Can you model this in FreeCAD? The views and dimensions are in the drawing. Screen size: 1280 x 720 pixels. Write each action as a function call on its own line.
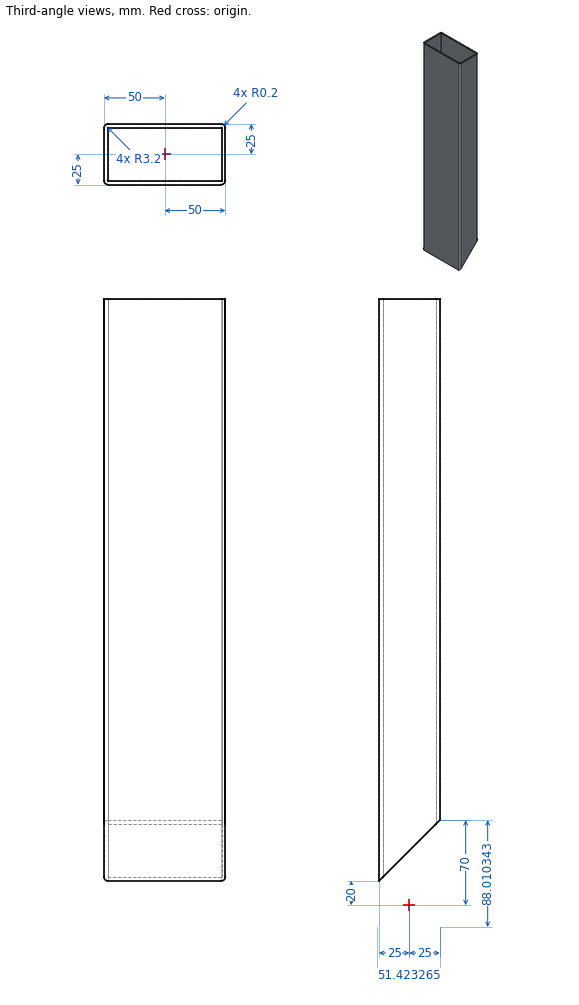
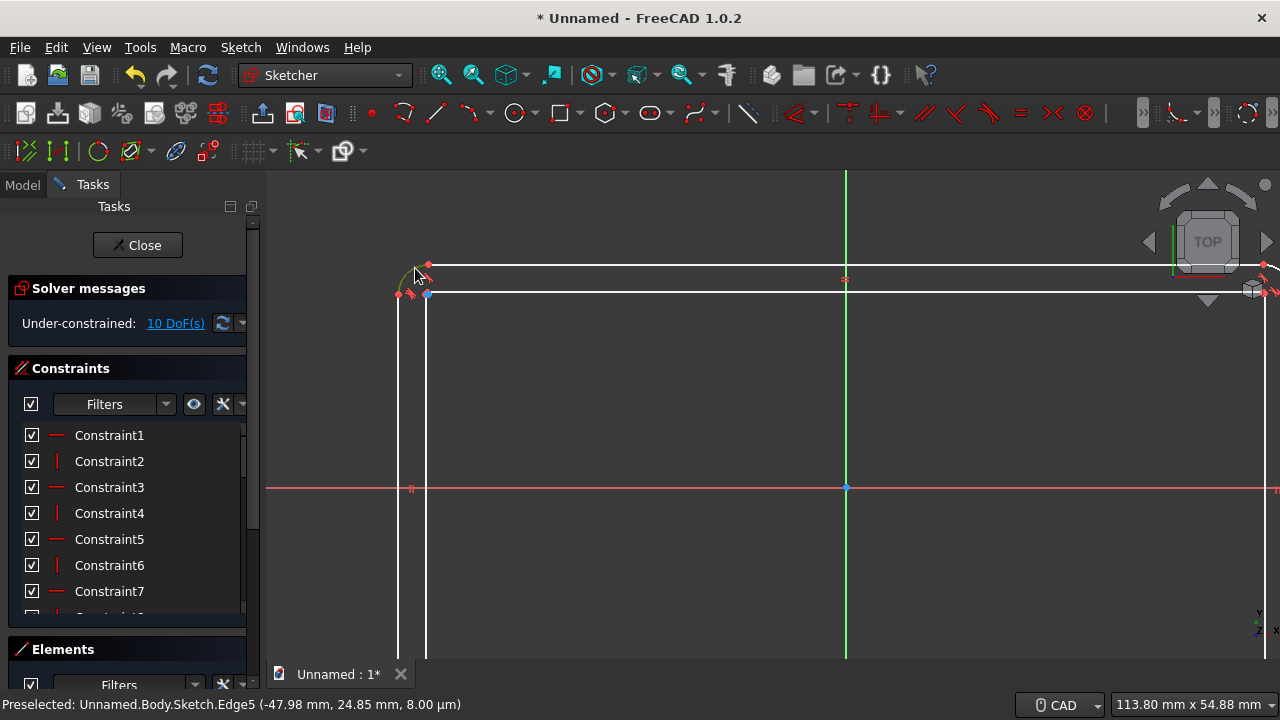
scroll(416, 265, down, 2)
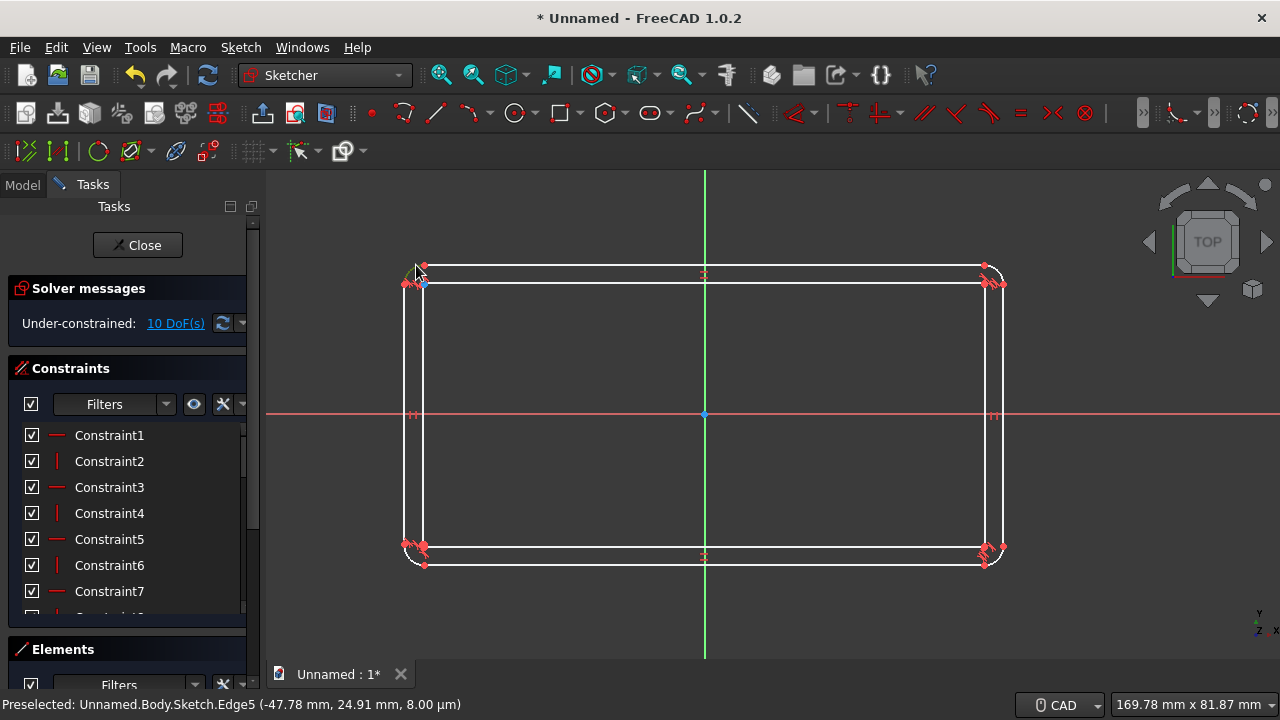
scroll(407, 554, up, 2)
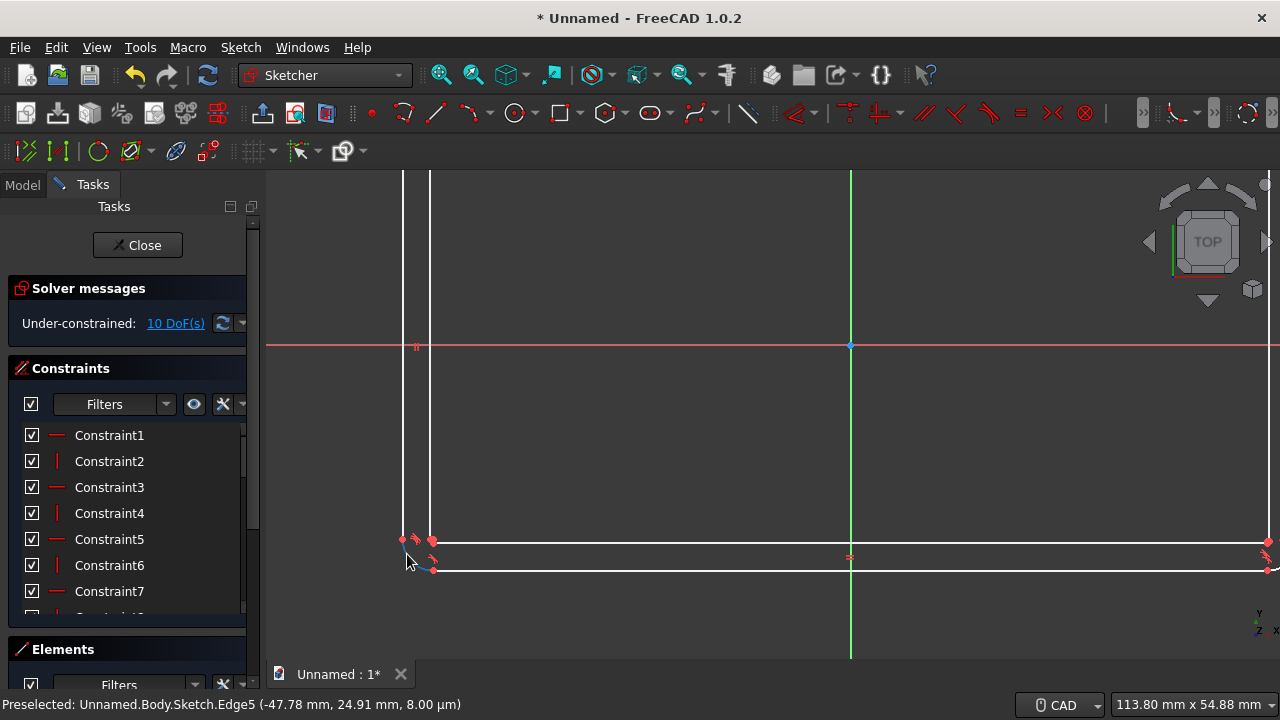
click(406, 554)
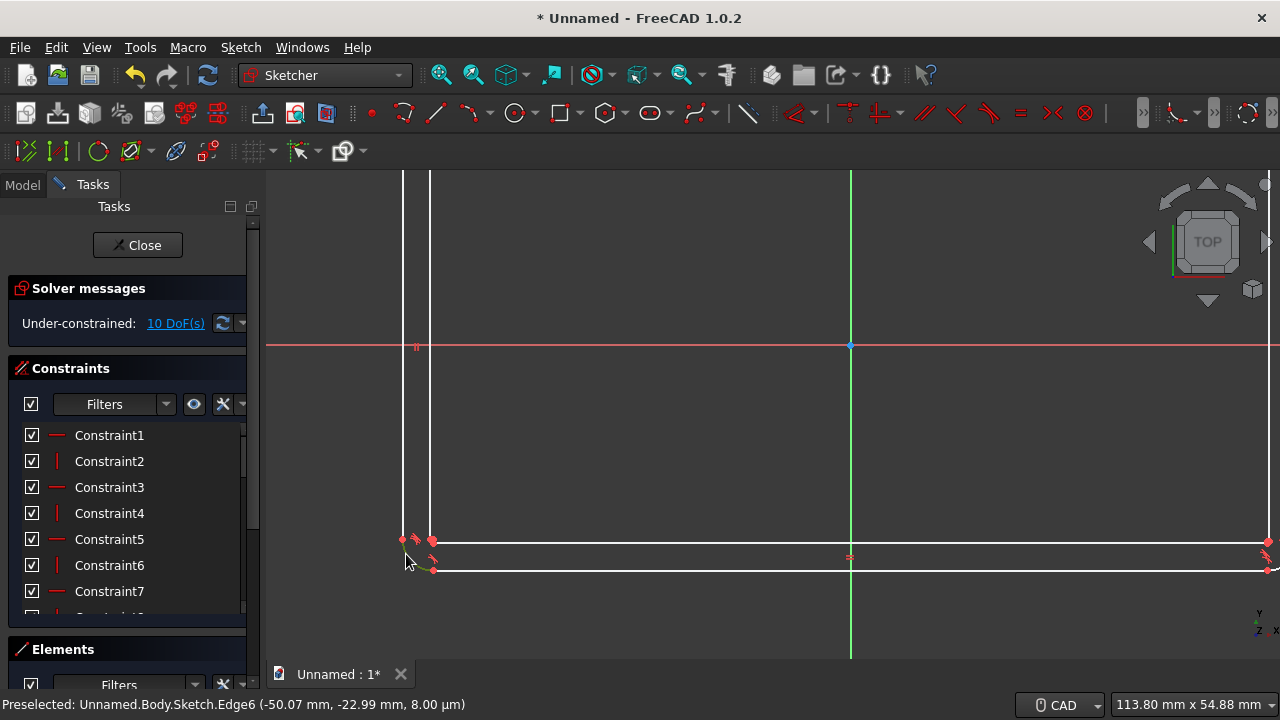
scroll(407, 555, down, 2)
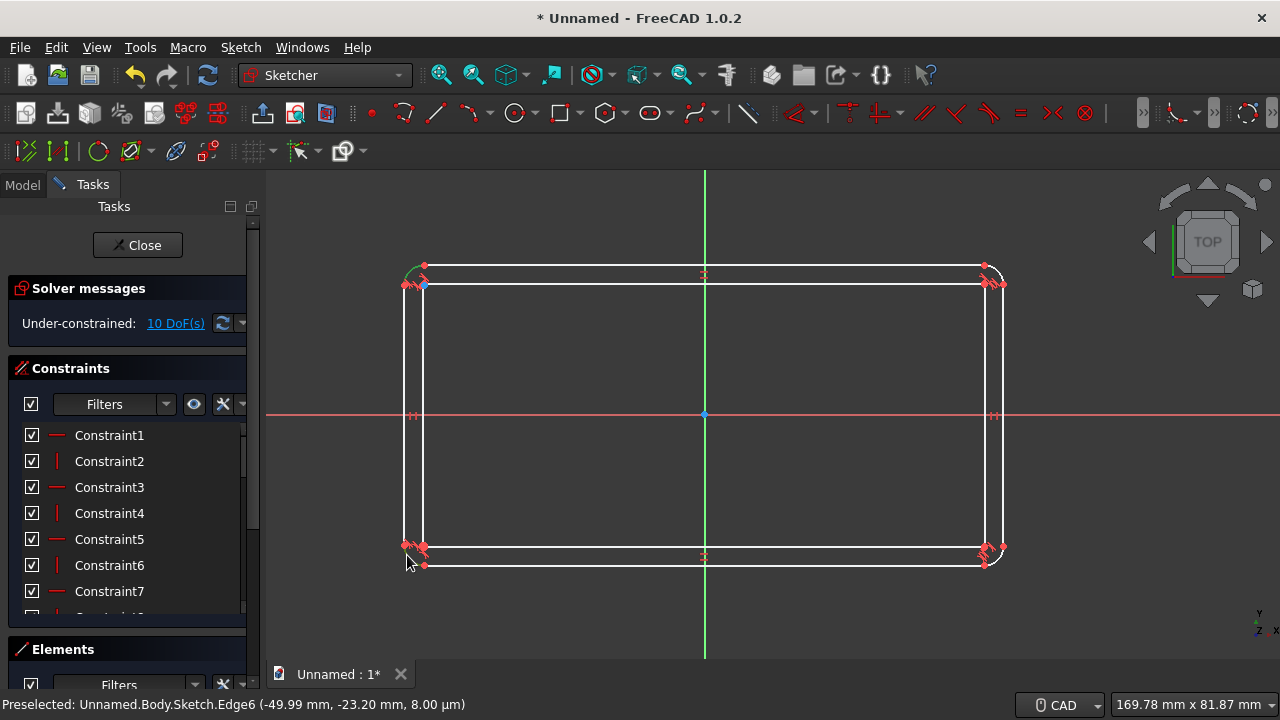
scroll(993, 564, up, 3)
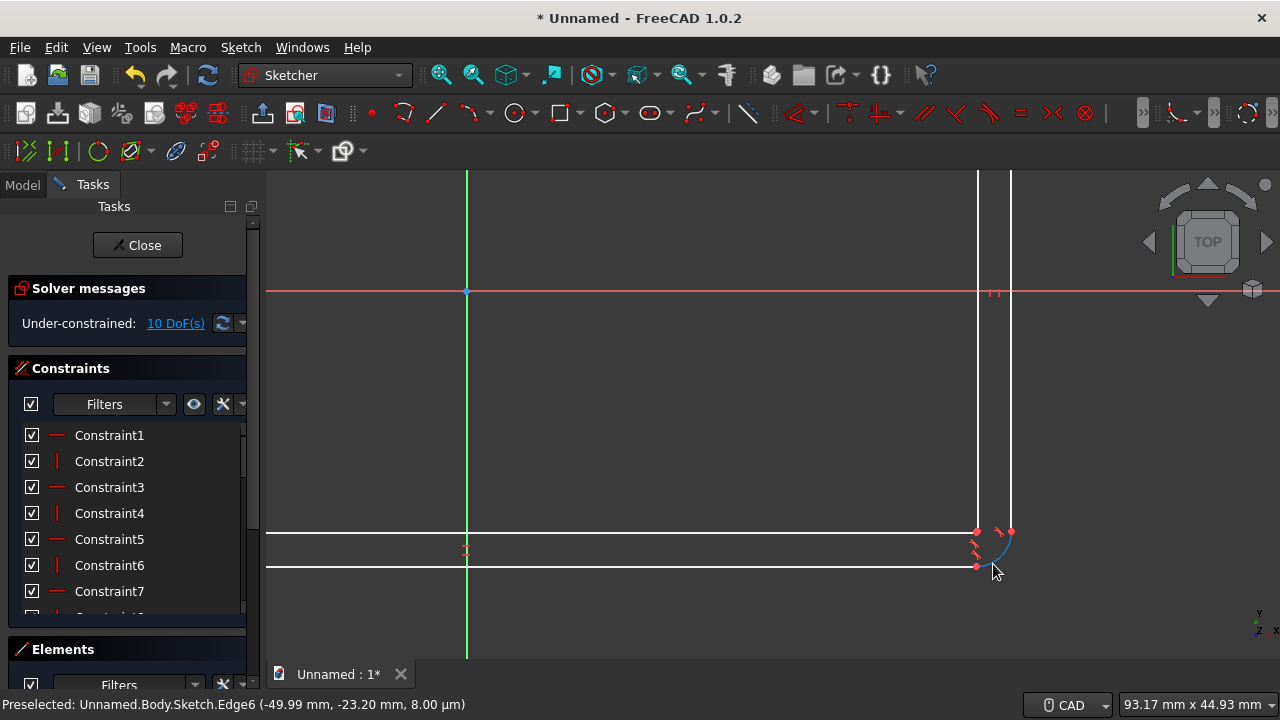
click(992, 563)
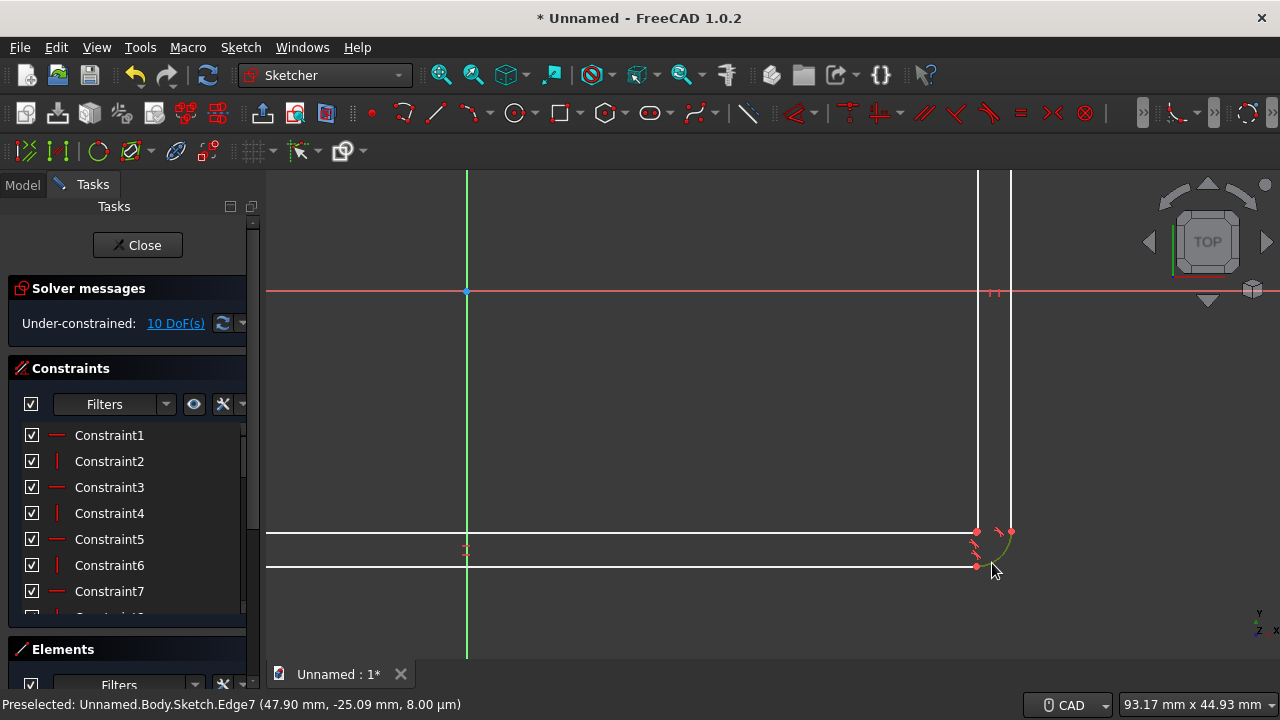
scroll(994, 564, down, 3)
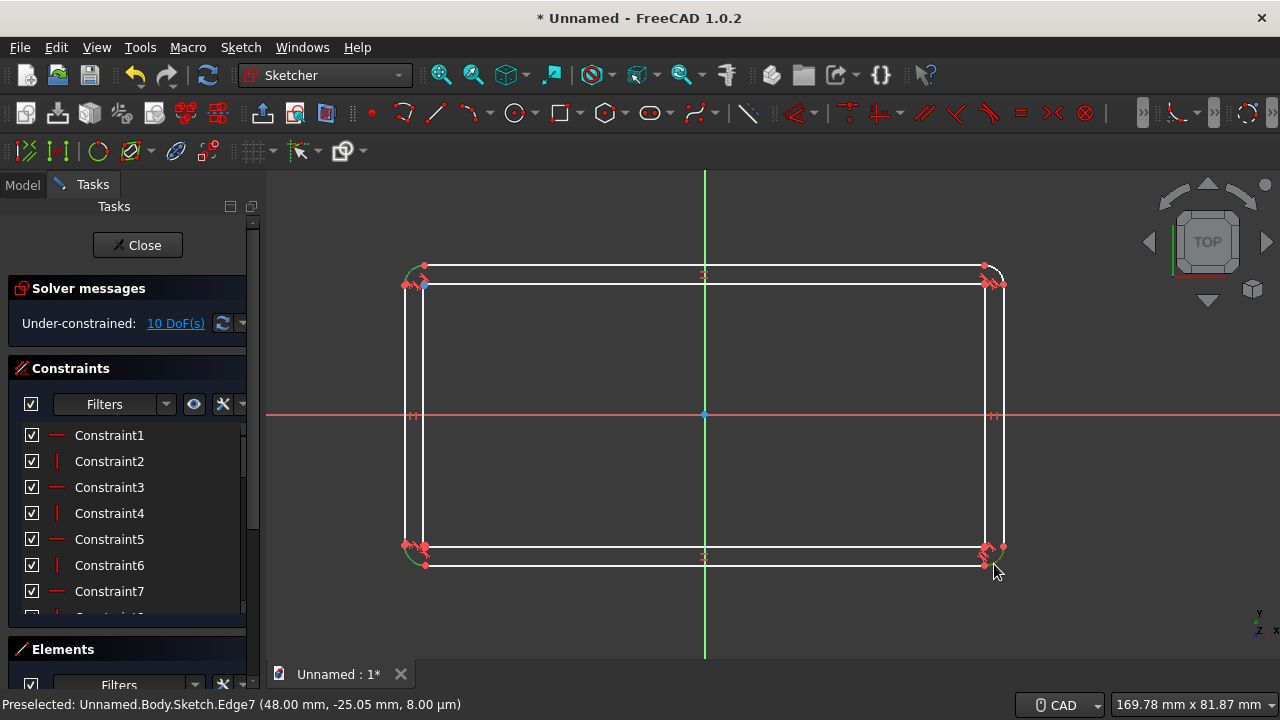
scroll(1002, 276, up, 3)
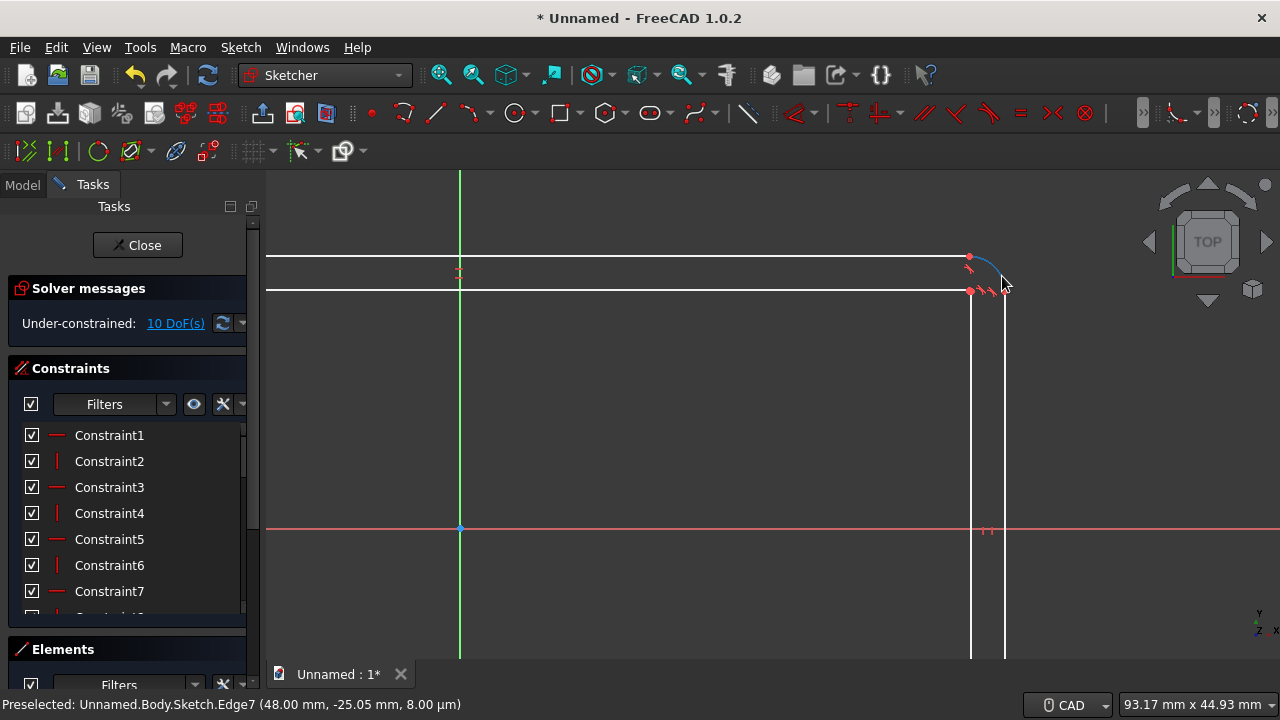
click(1001, 276)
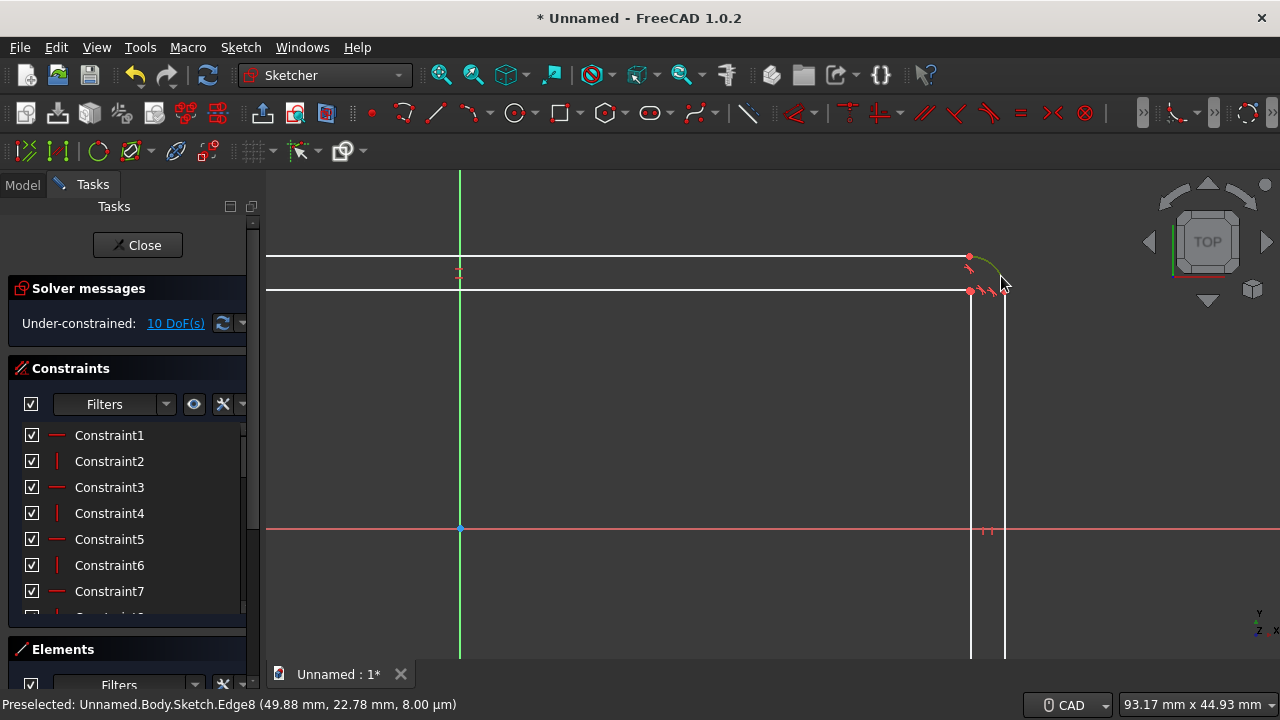
click(1022, 114)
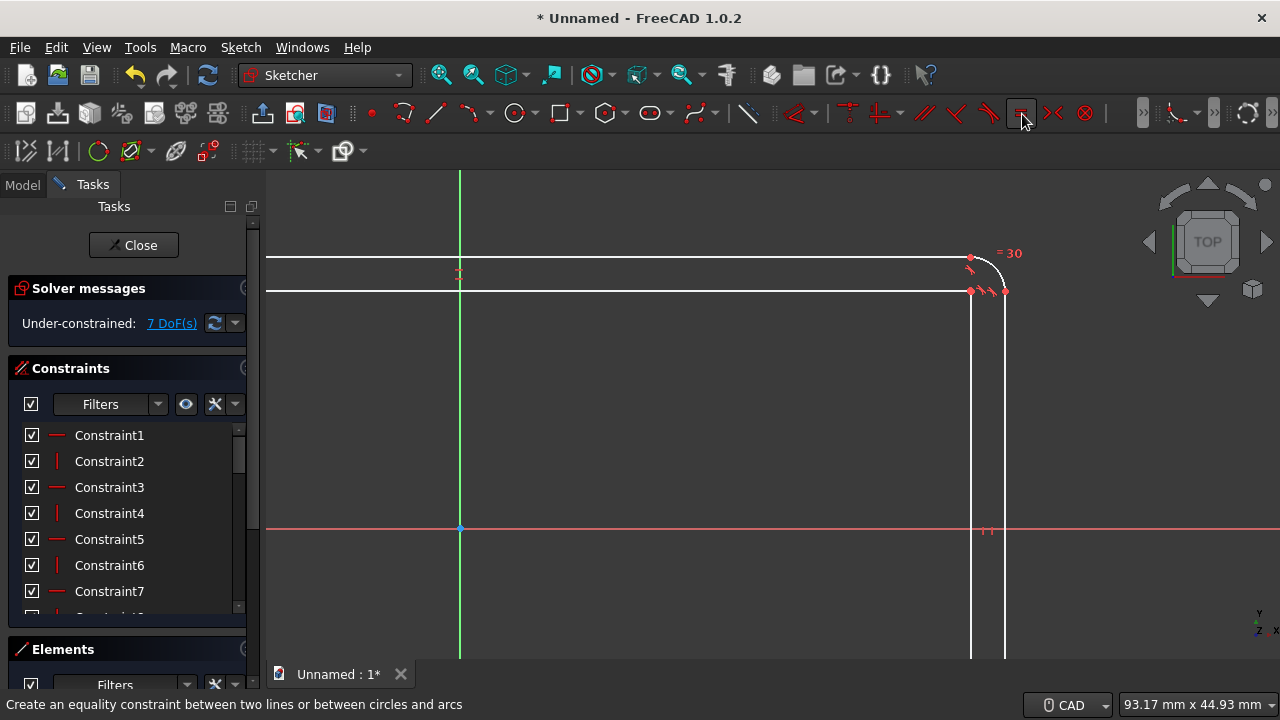
scroll(971, 291, up, 10)